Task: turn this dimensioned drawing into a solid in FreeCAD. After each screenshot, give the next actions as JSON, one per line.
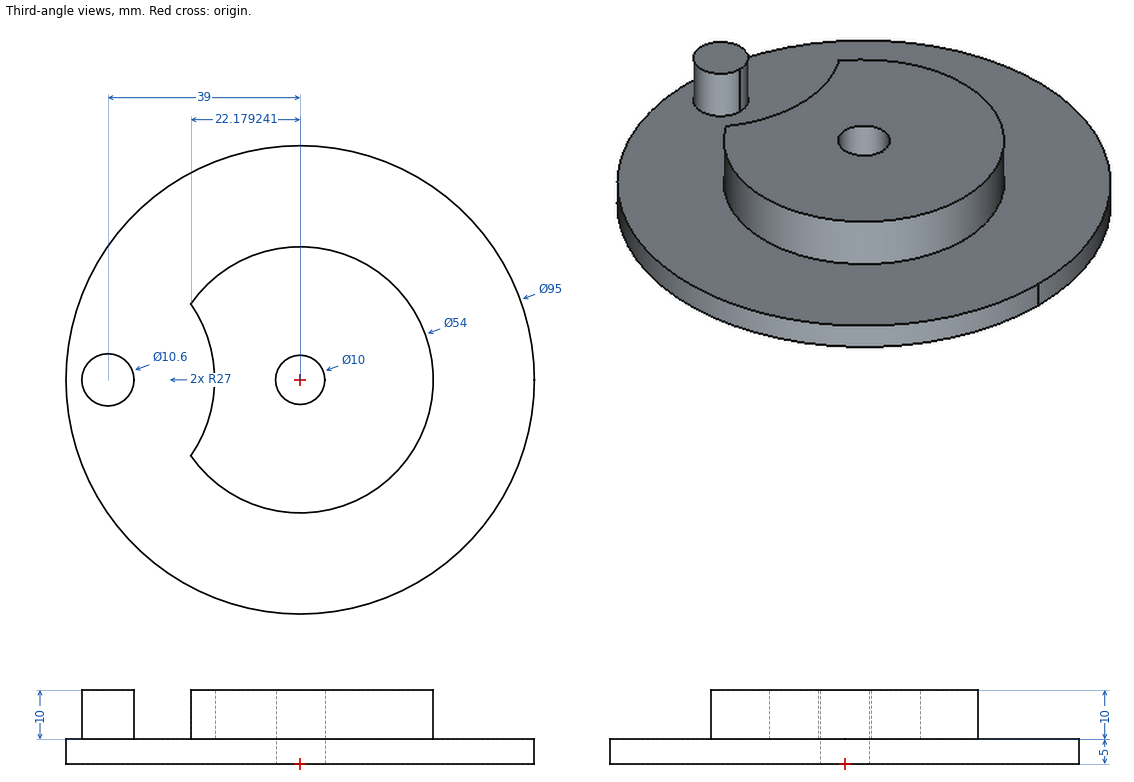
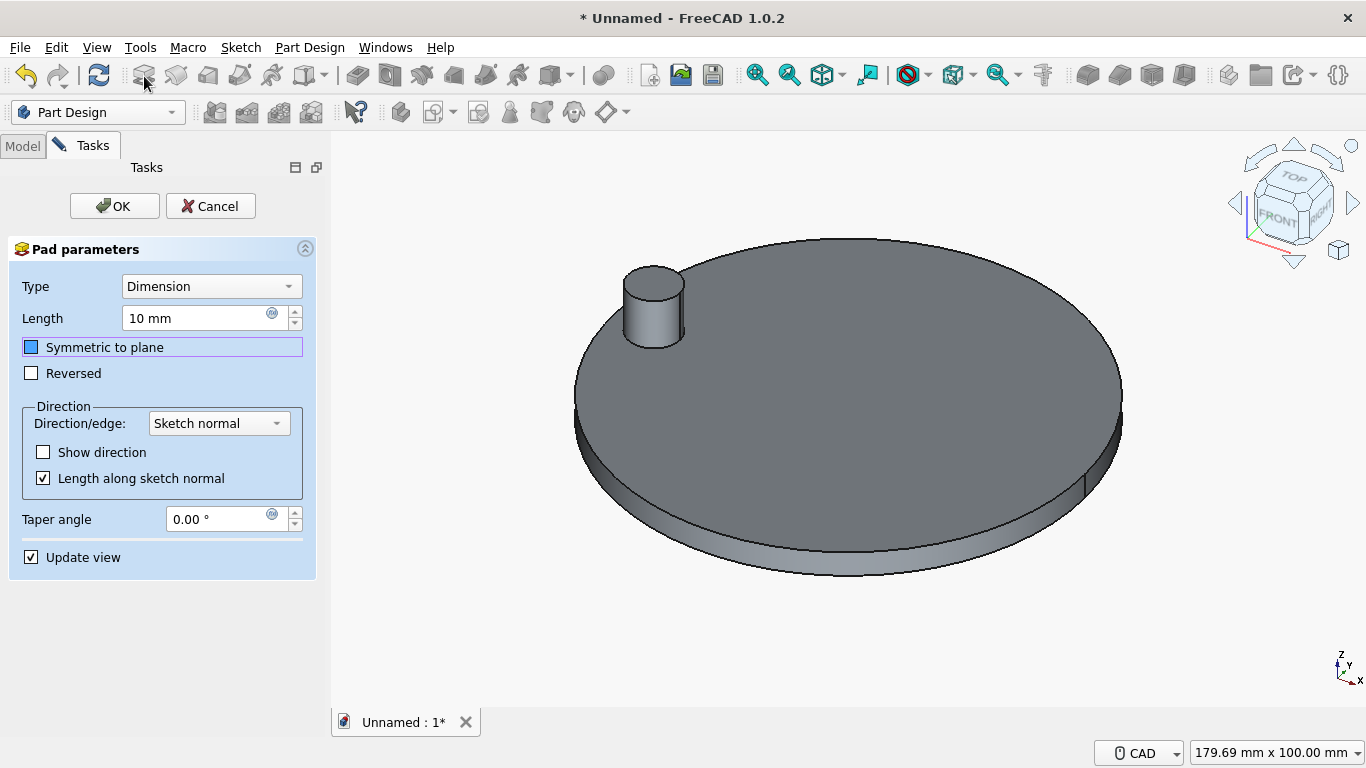
{"action": "left_click", "coordinate": [115, 206]}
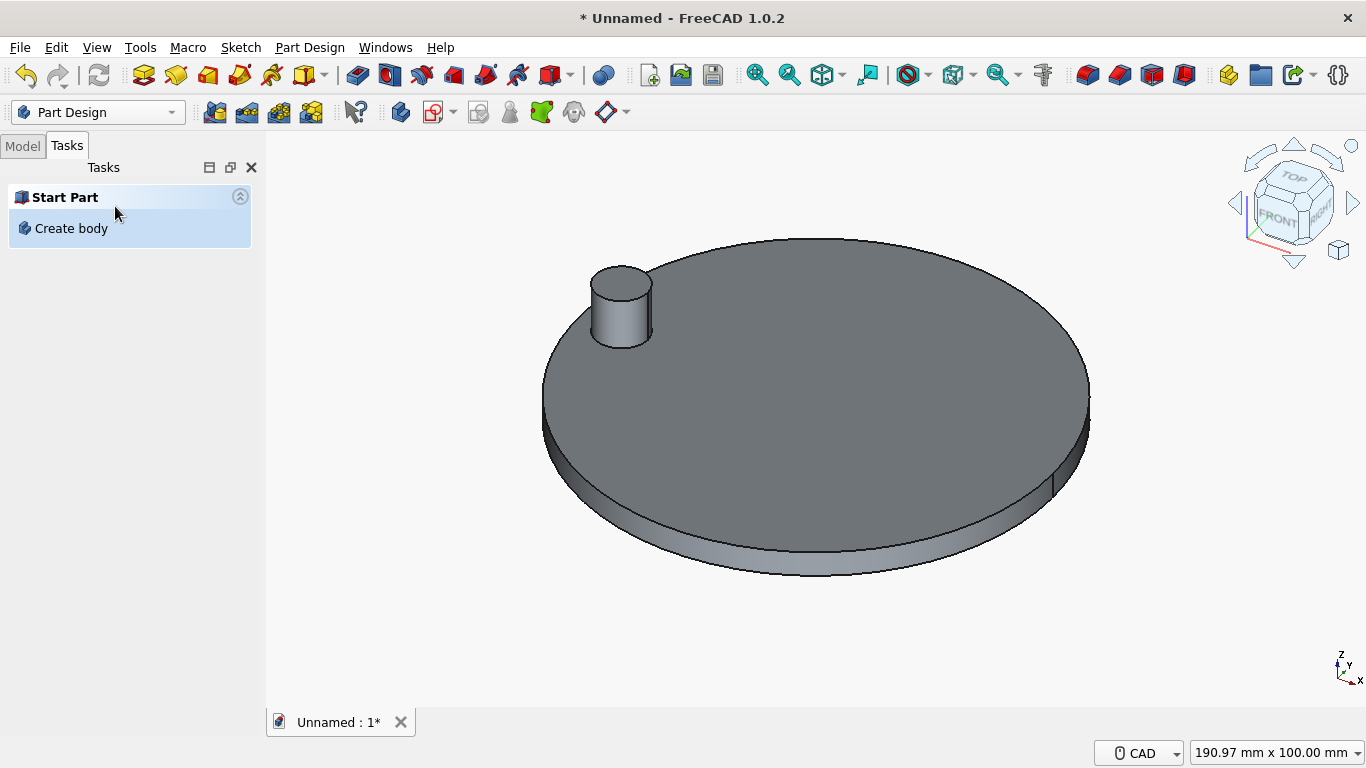
{"action": "left_click", "coordinate": [884, 417]}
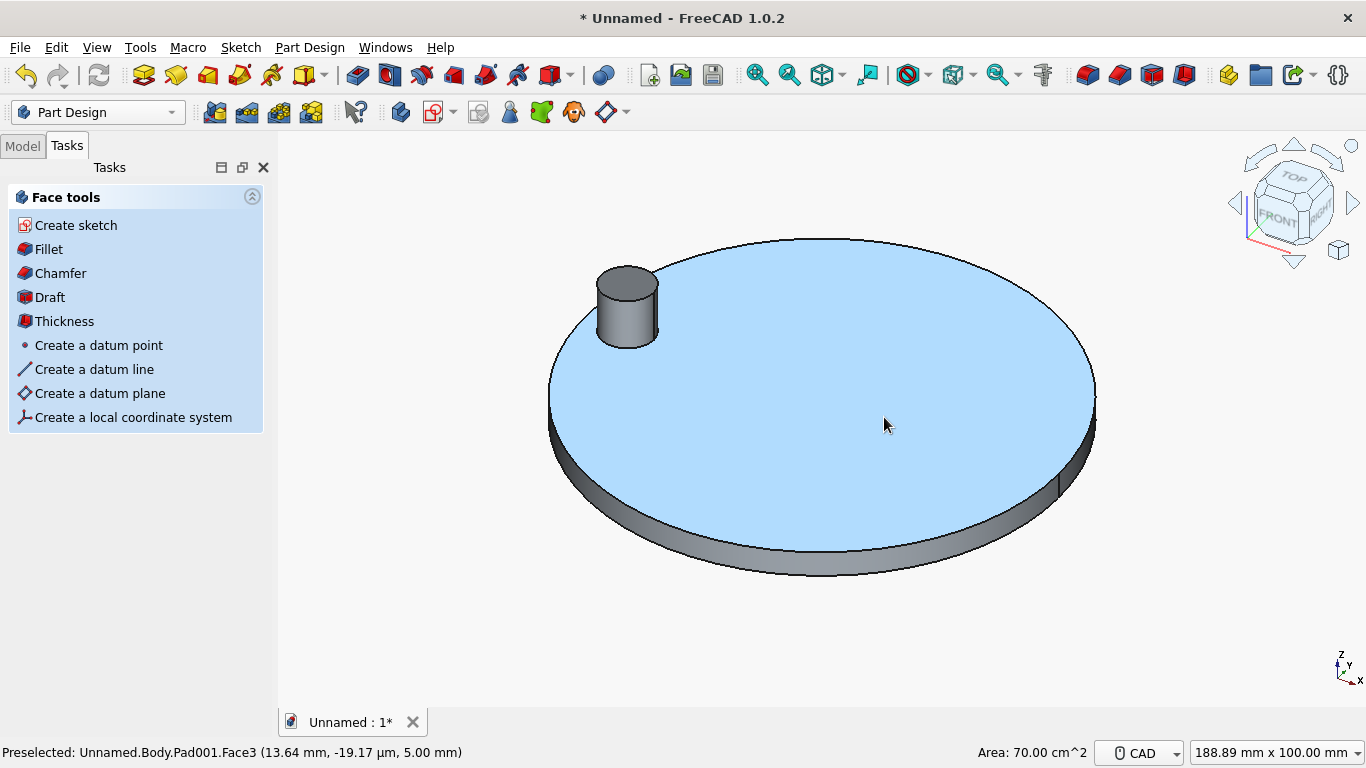
{"action": "left_click", "coordinate": [434, 112]}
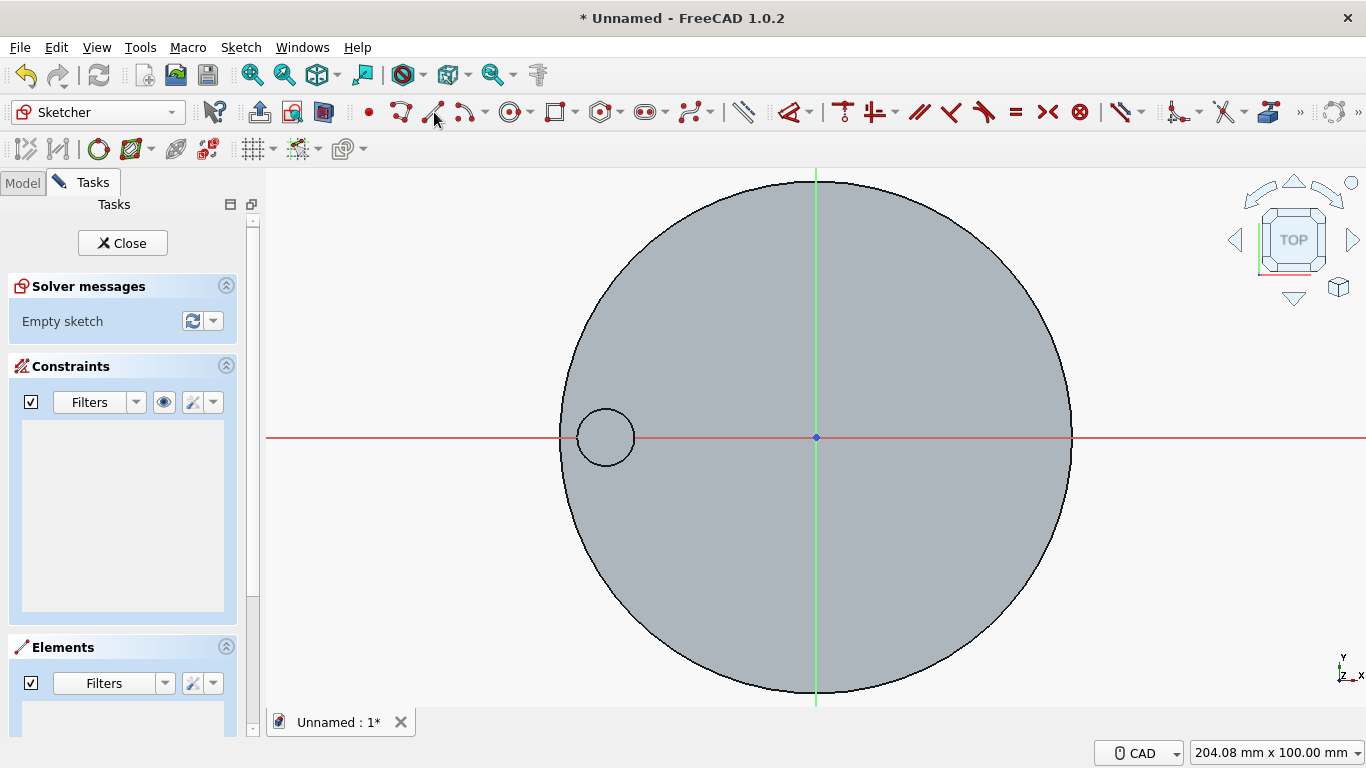
{"action": "key", "text": "q s"}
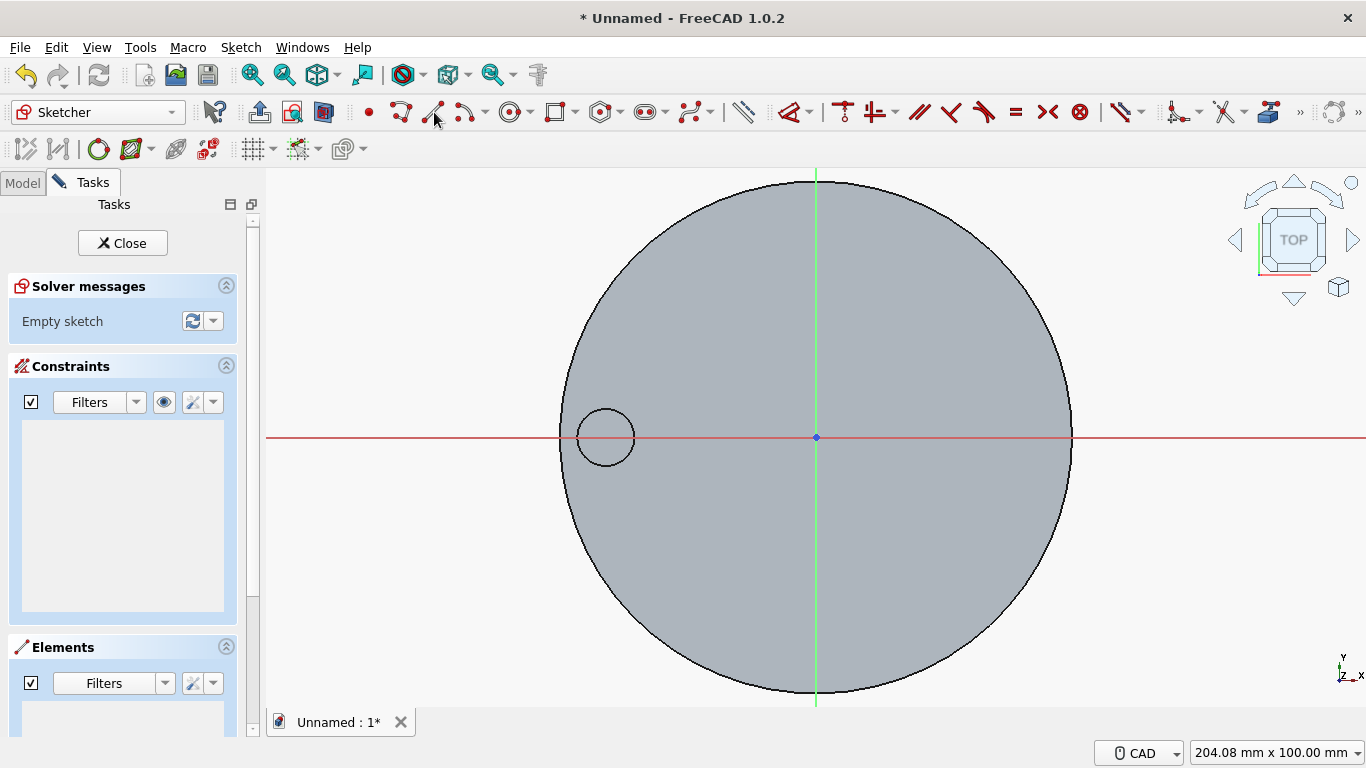
{"action": "key", "text": "g c"}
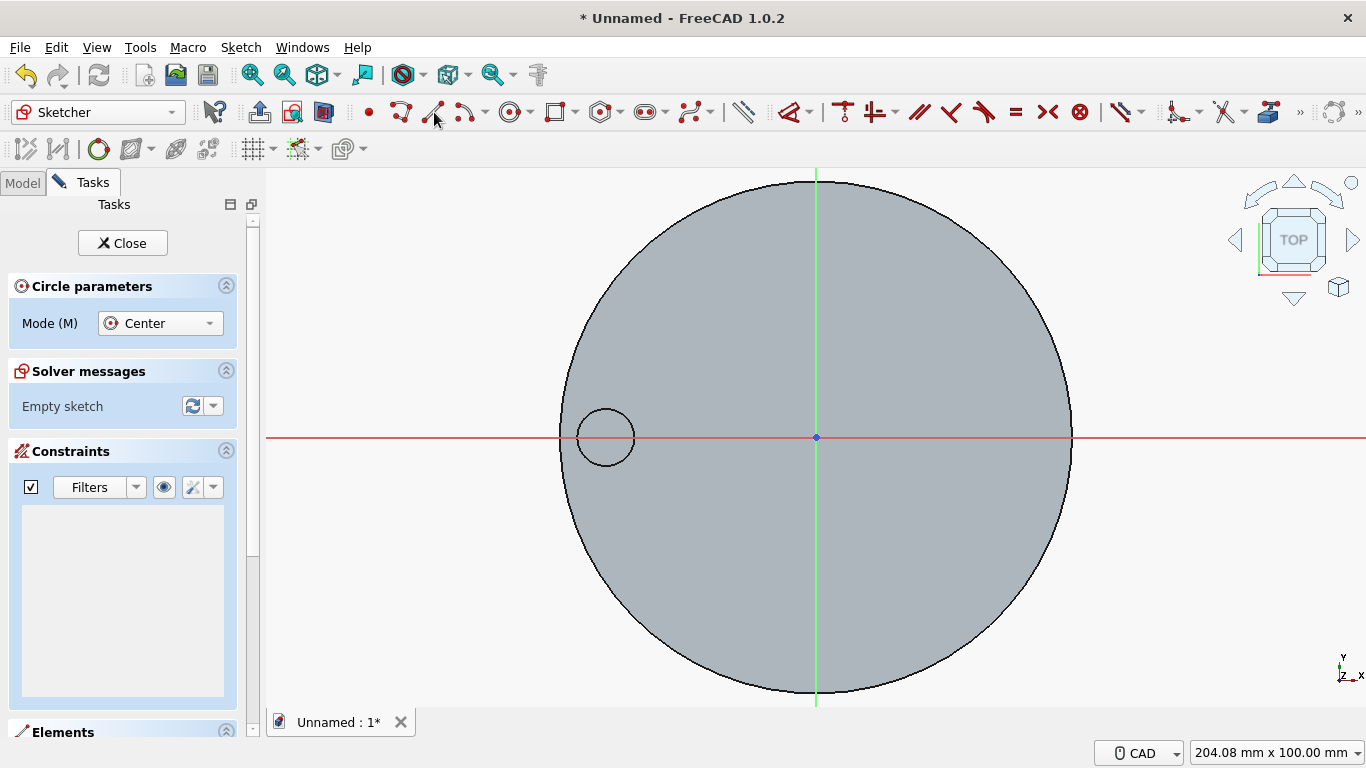
{"action": "left_click", "coordinate": [816, 438]}
{"action": "left_click", "coordinate": [919, 335]}
{"action": "key", "text": "Escape"}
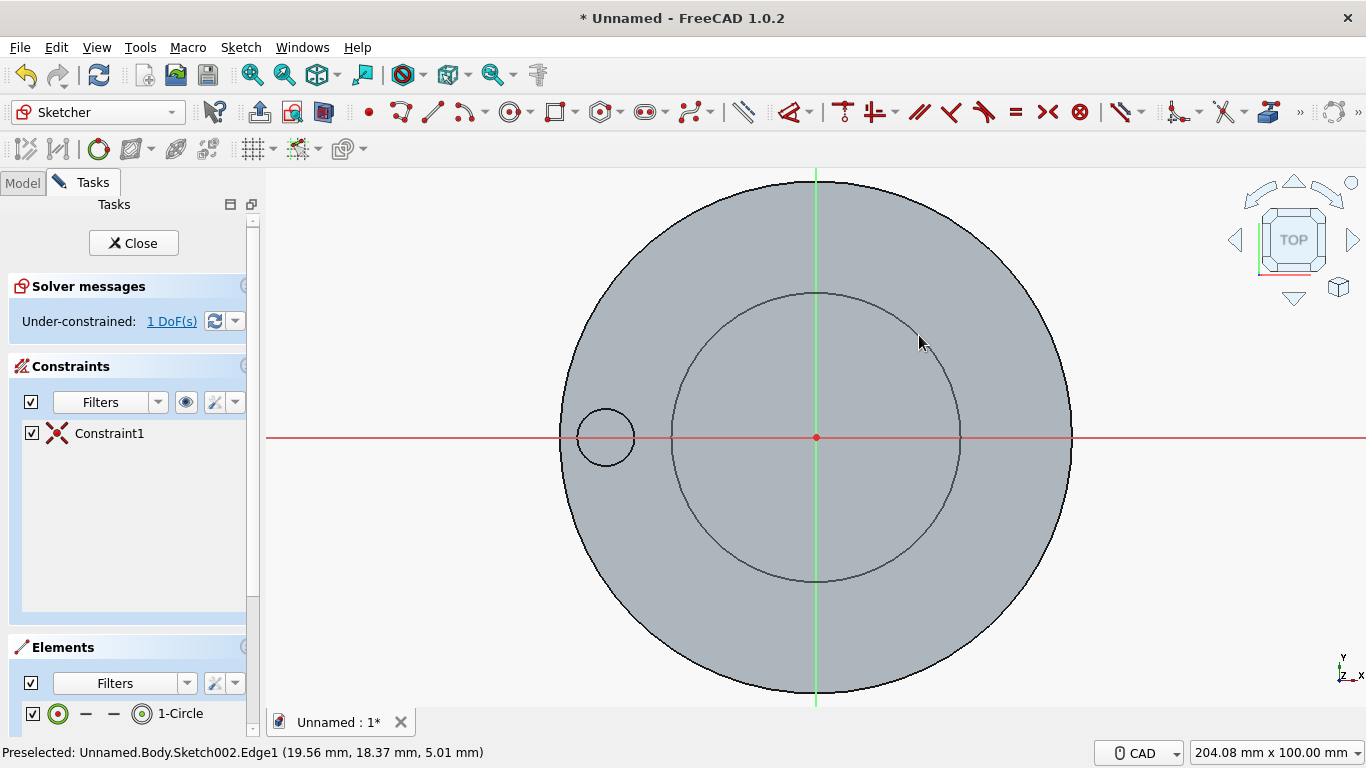
{"action": "key", "text": "d"}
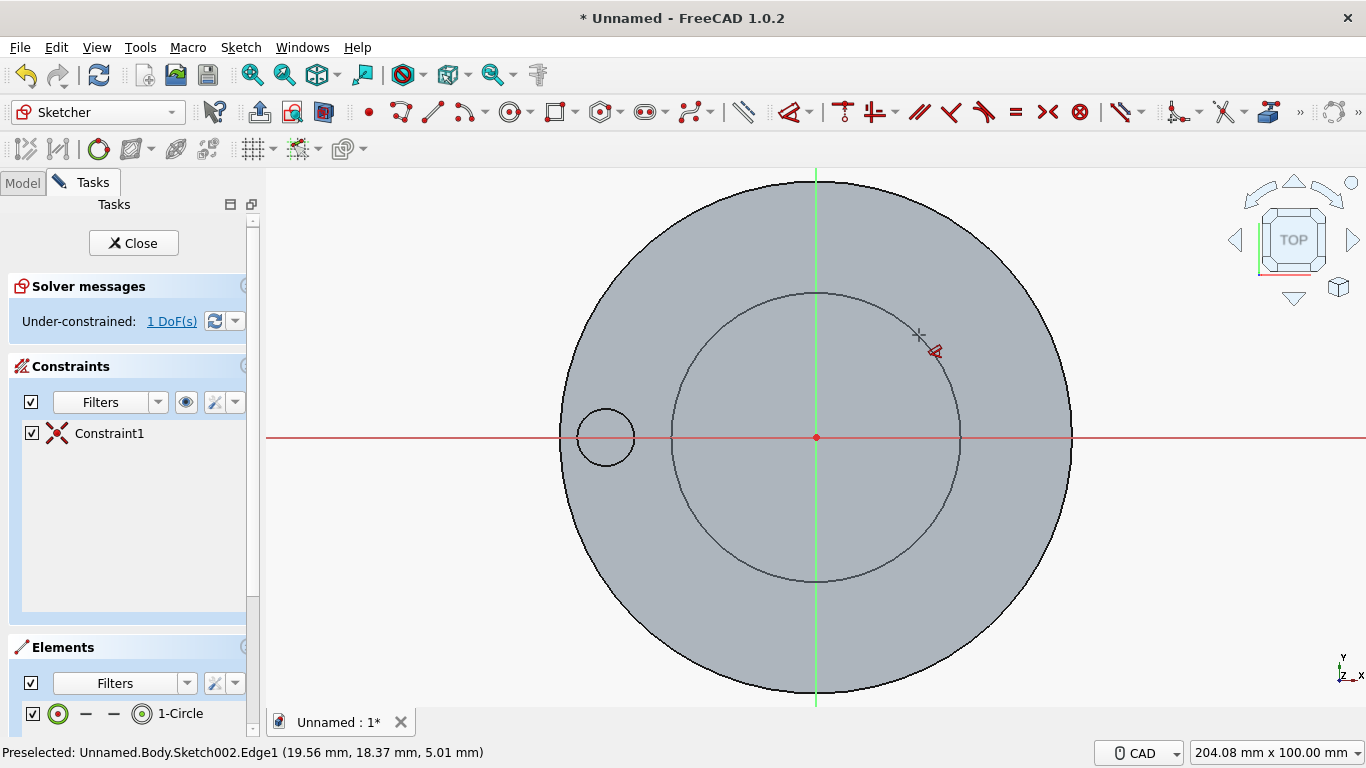
{"action": "left_click", "coordinate": [918, 335]}
{"action": "left_click", "coordinate": [941, 312]}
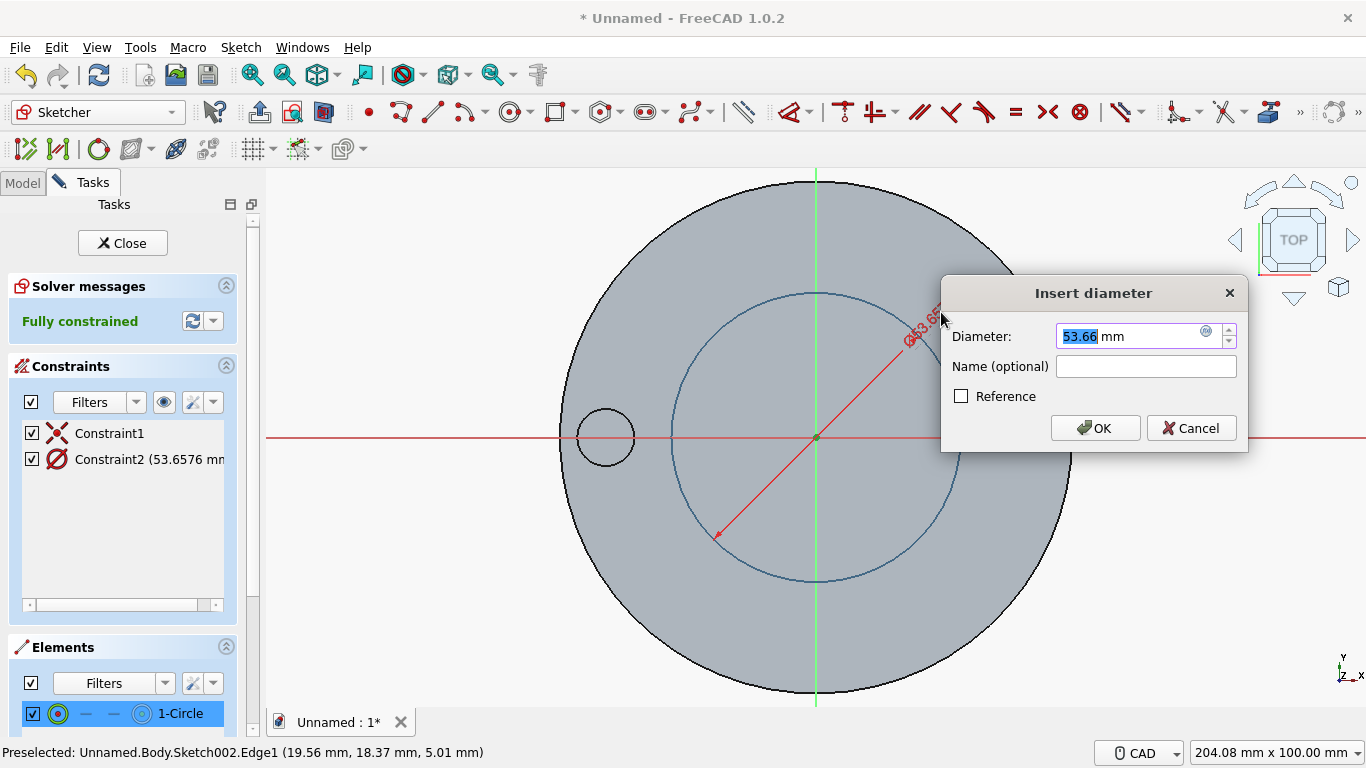
{"action": "type", "text": "54"}
{"action": "key", "text": "Return"}
{"action": "key", "text": "Escape"}